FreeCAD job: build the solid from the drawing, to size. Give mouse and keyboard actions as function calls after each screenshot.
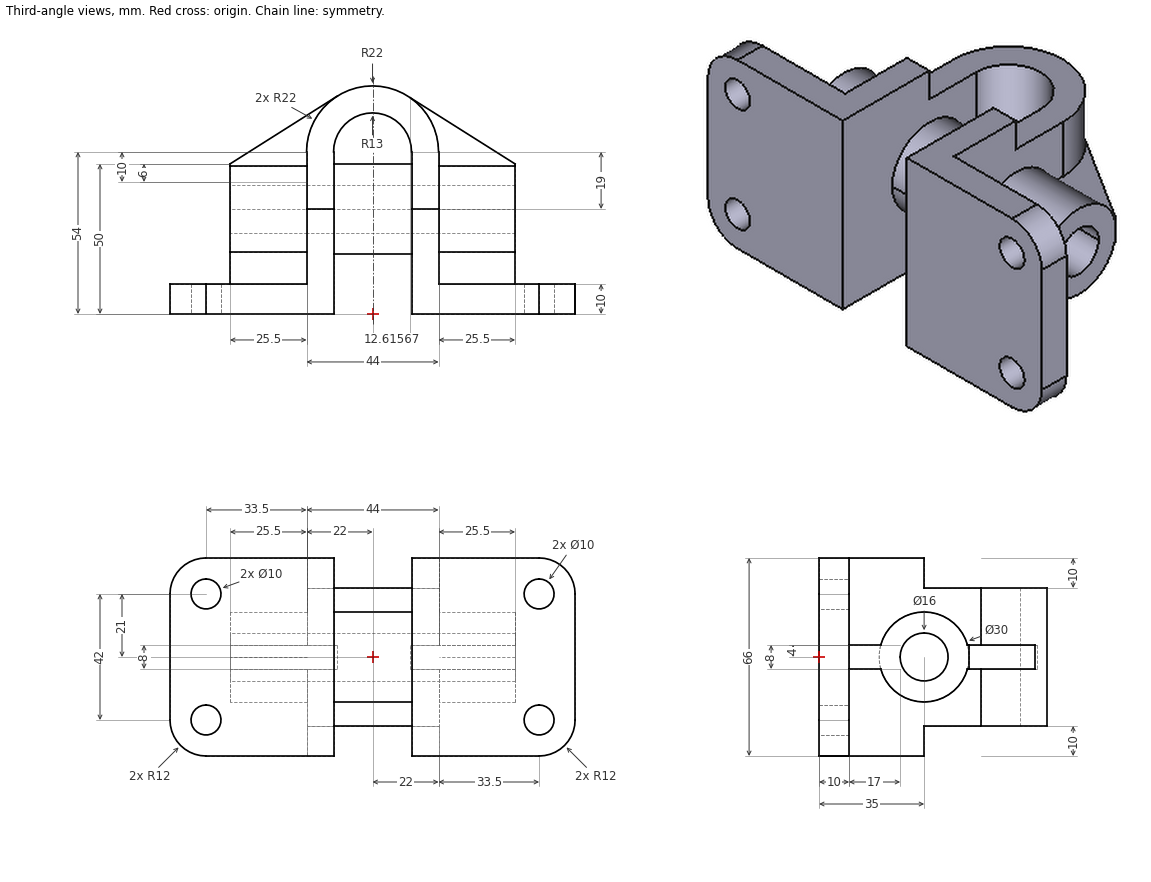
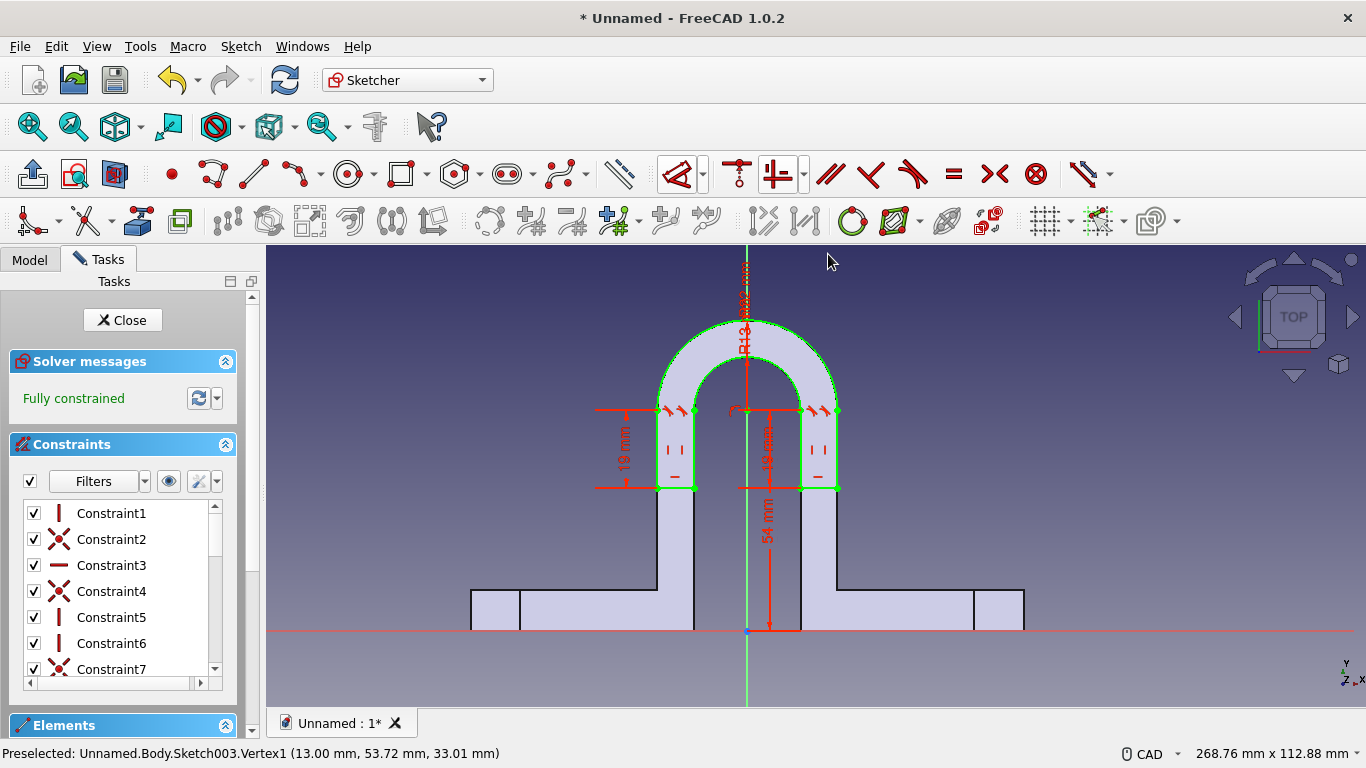
click(123, 320)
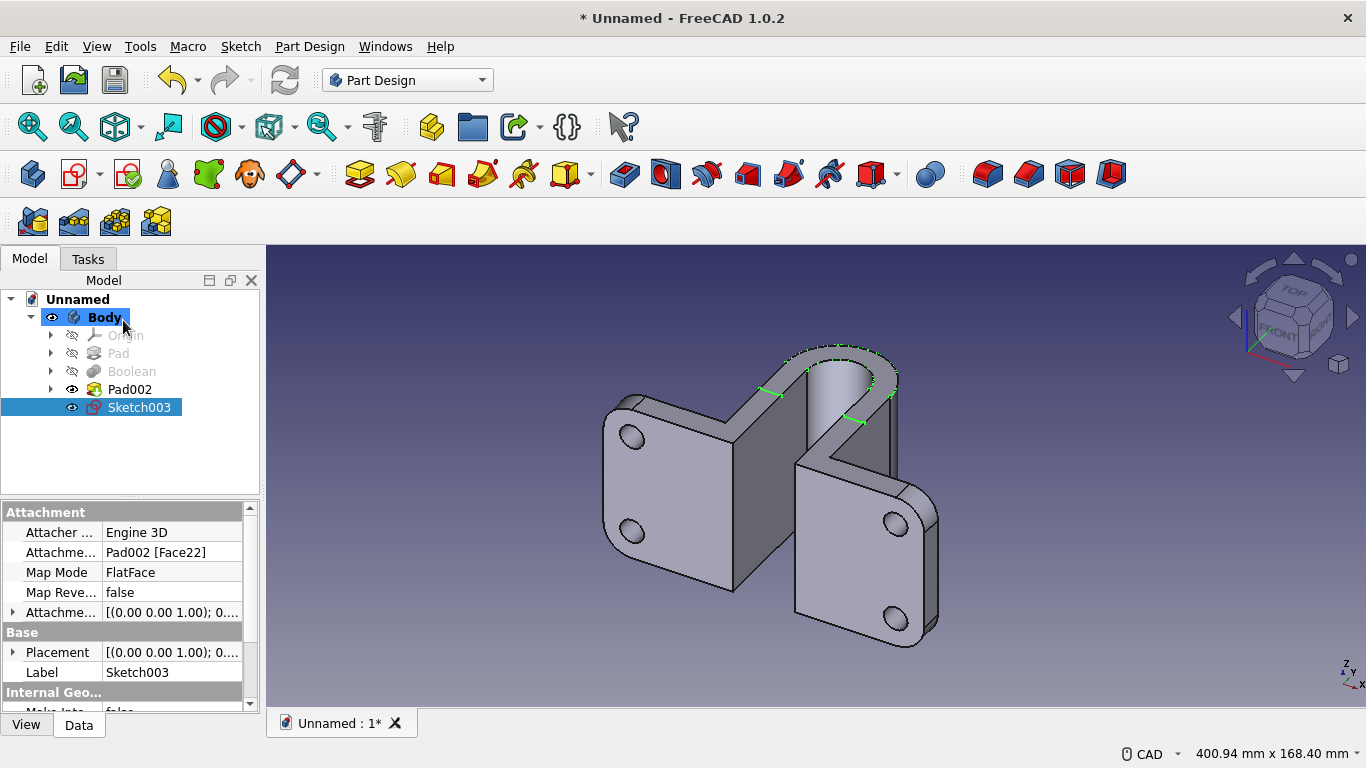
click(625, 174)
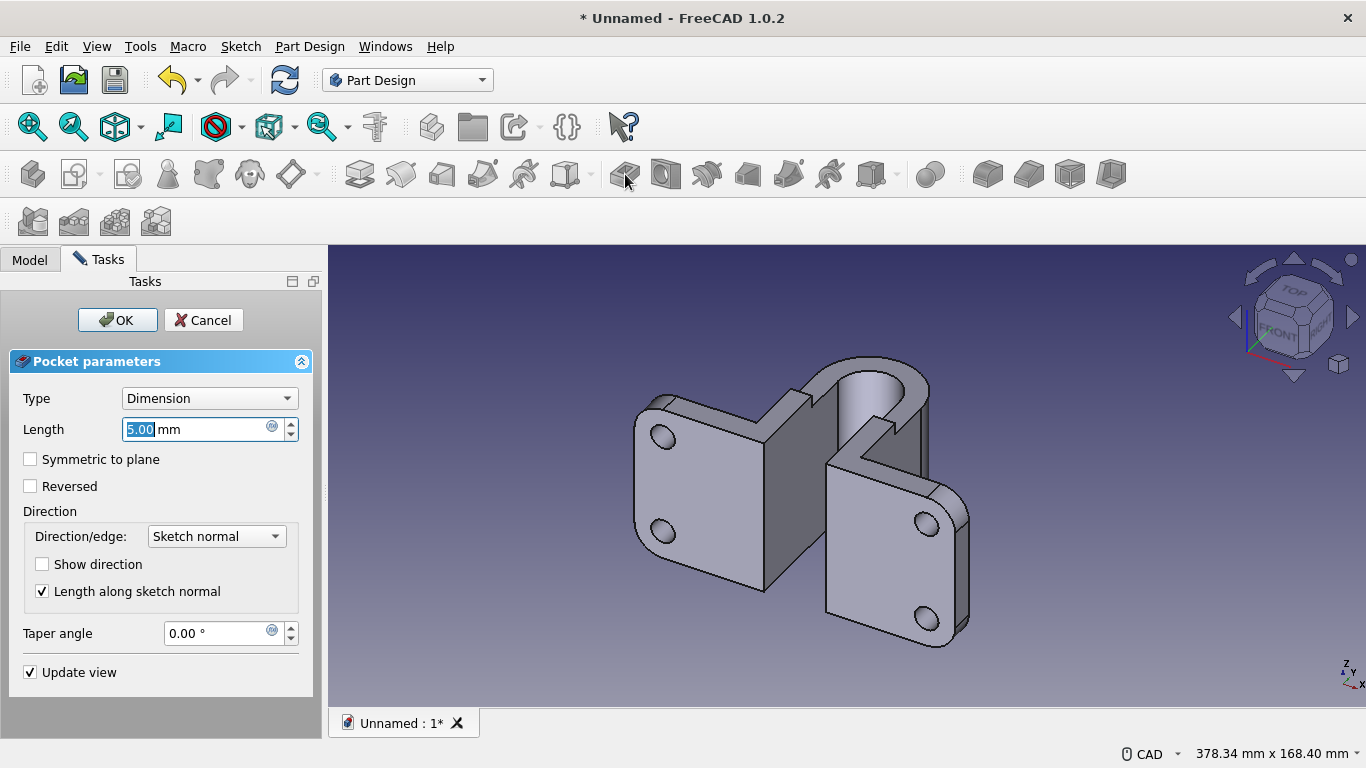
text(10)
key(Tab)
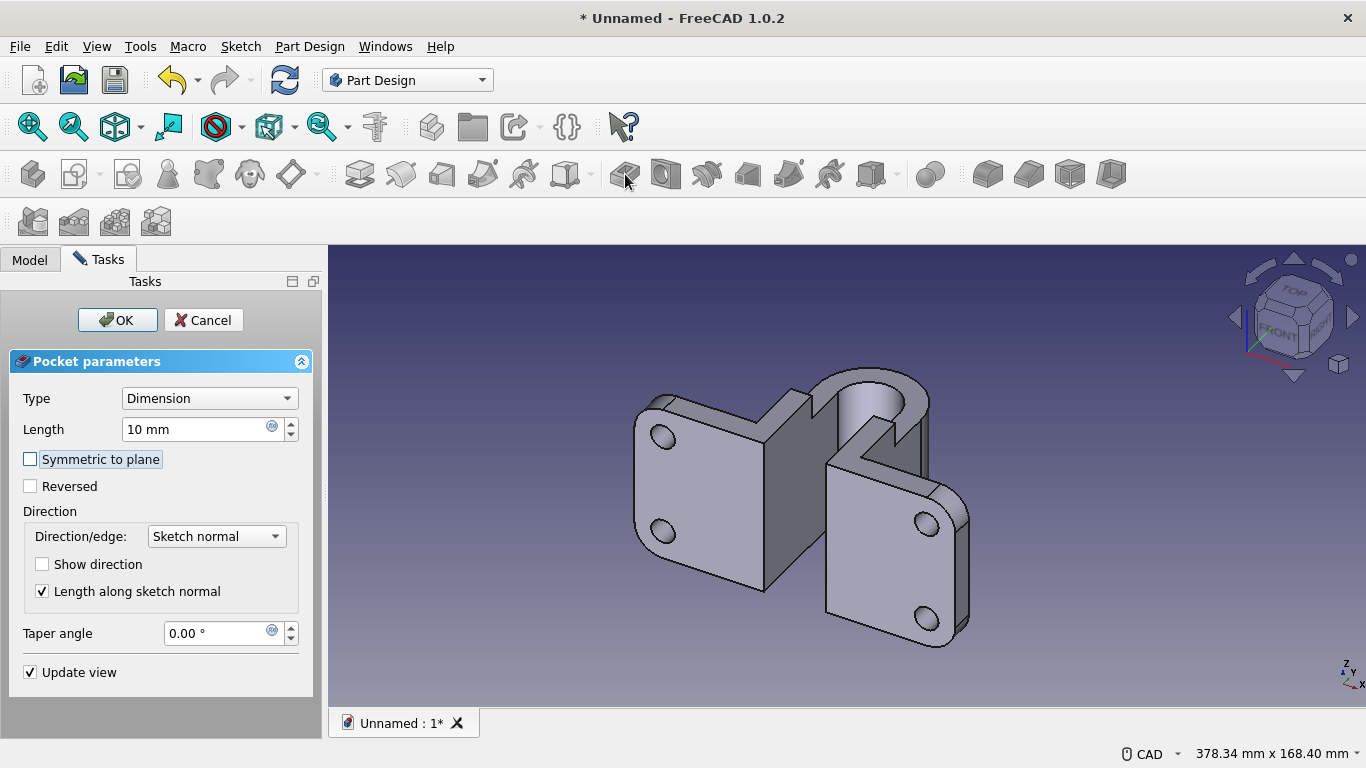
click(118, 320)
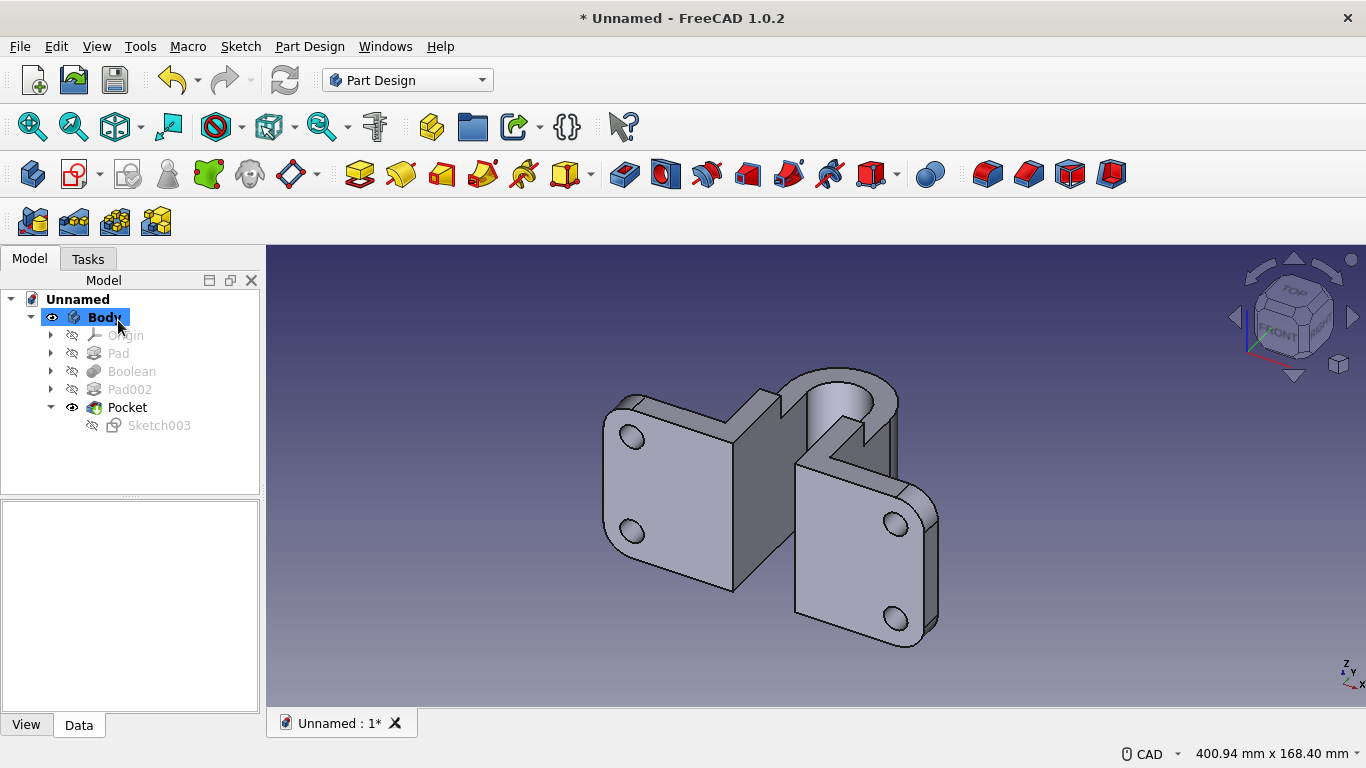
click(51, 335)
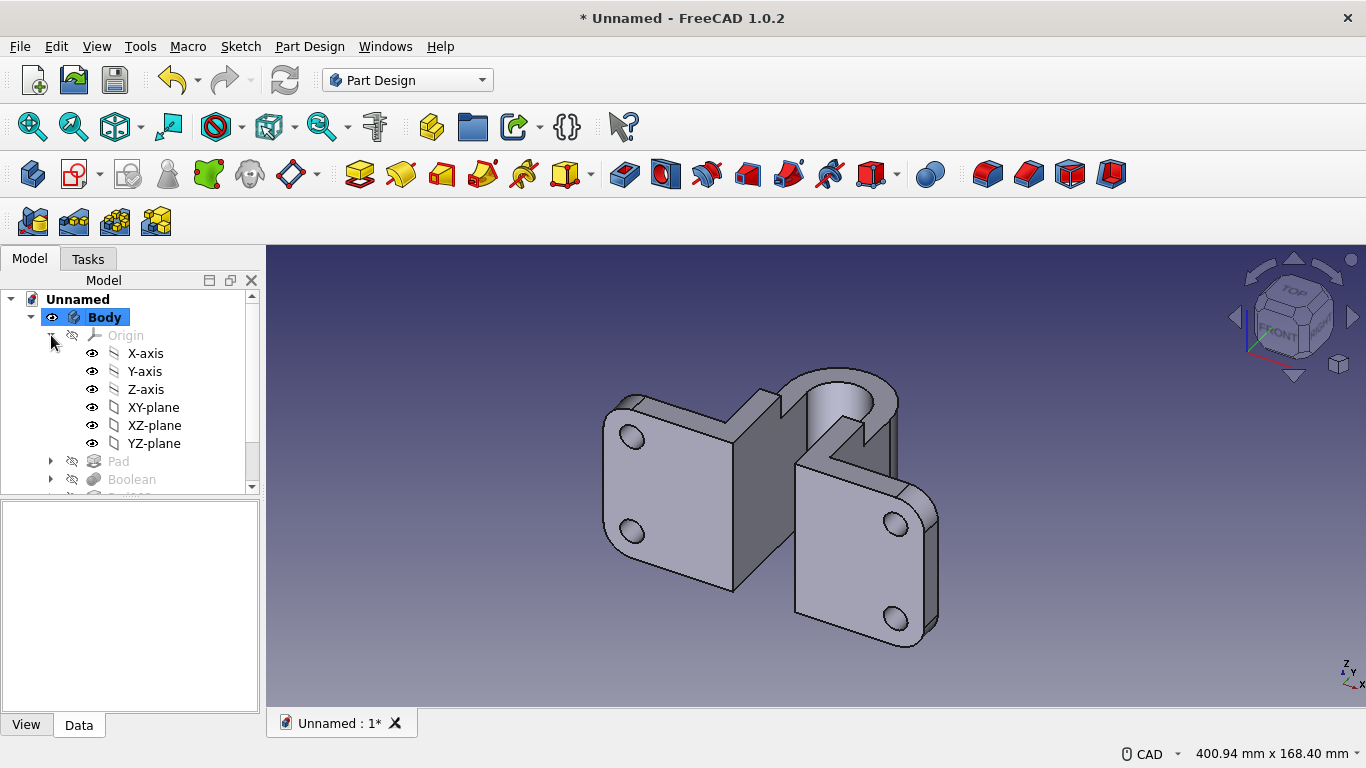
click(137, 407)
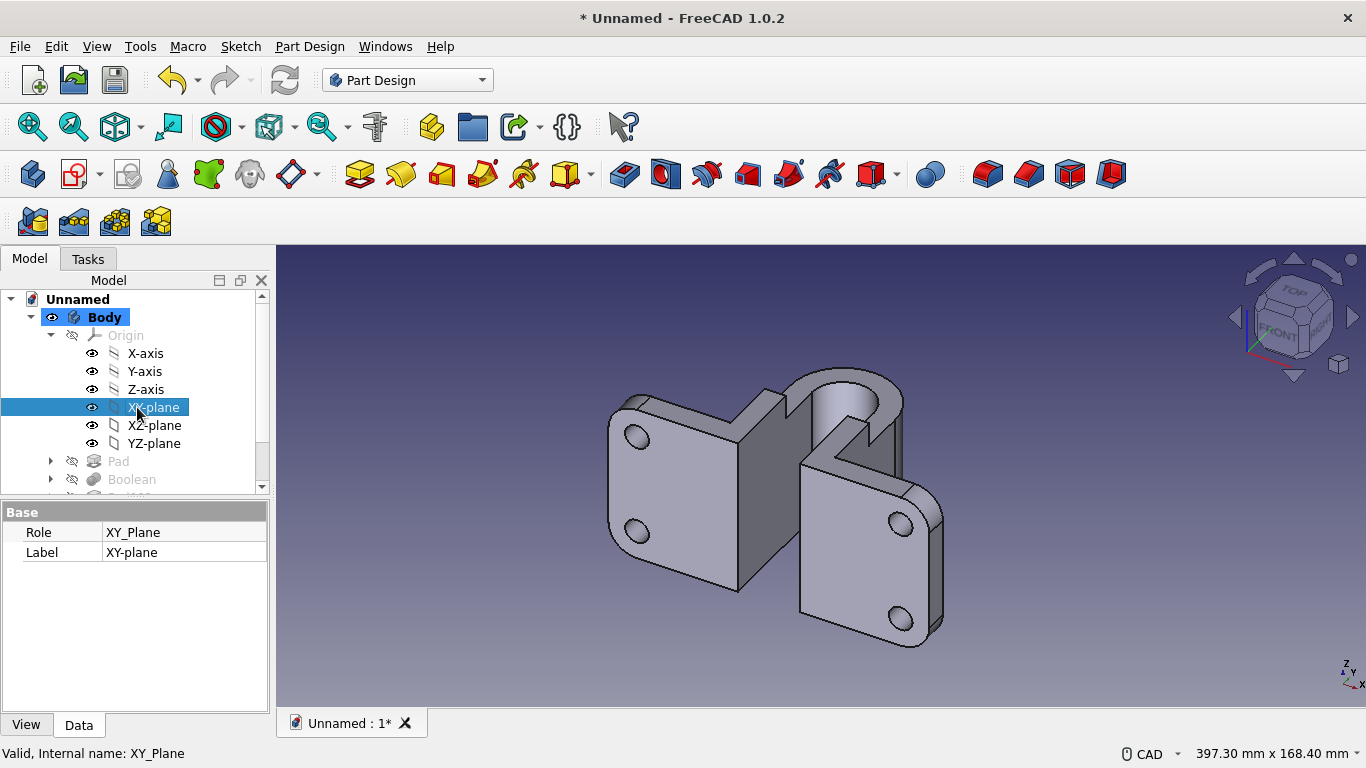
click(290, 174)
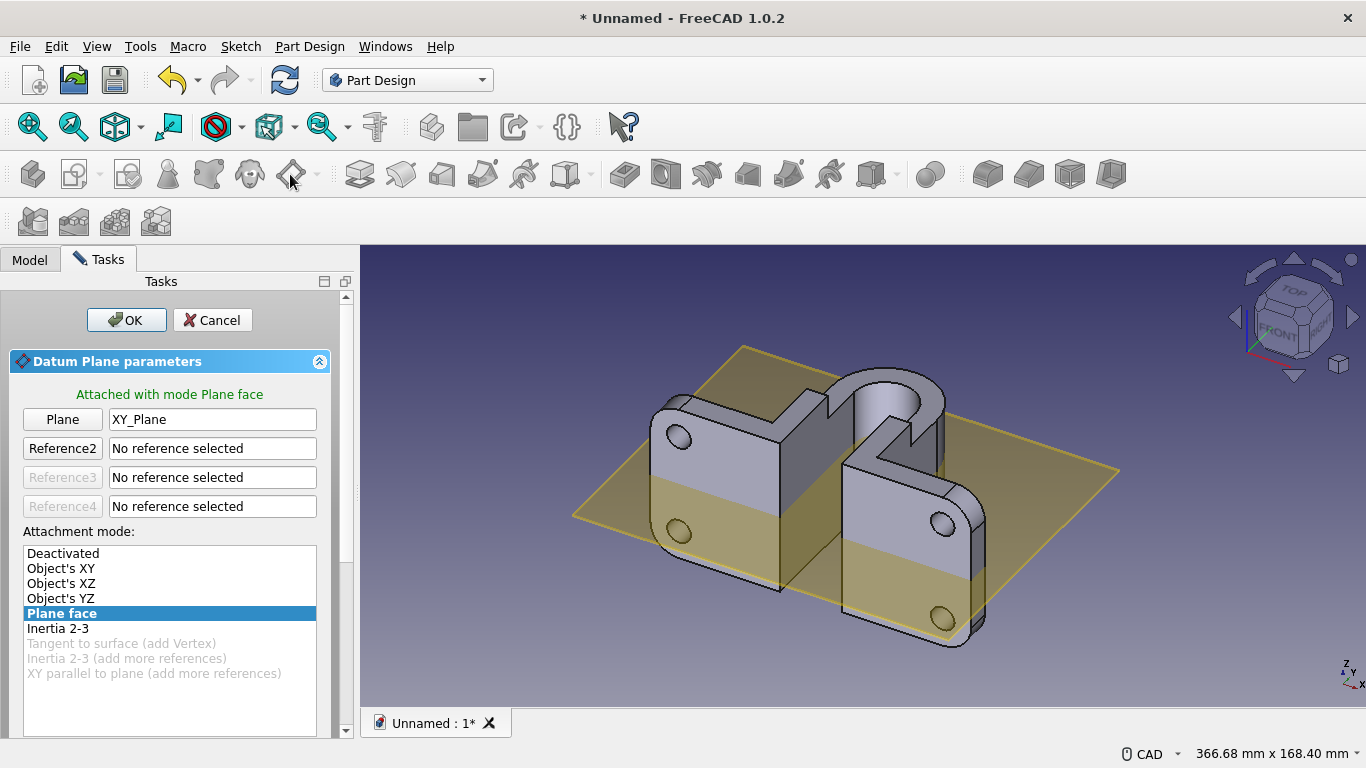
scroll(346, 514, down, 4)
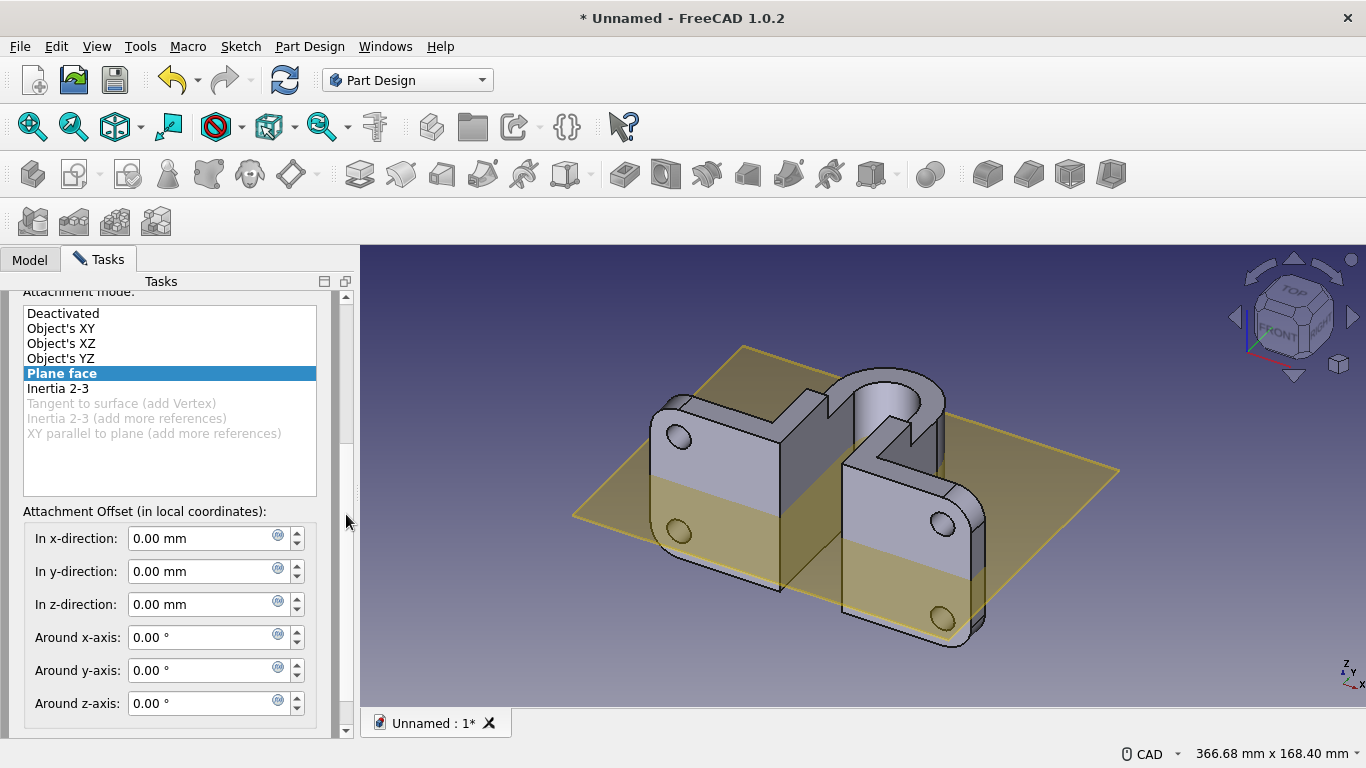
triple_click(210, 604)